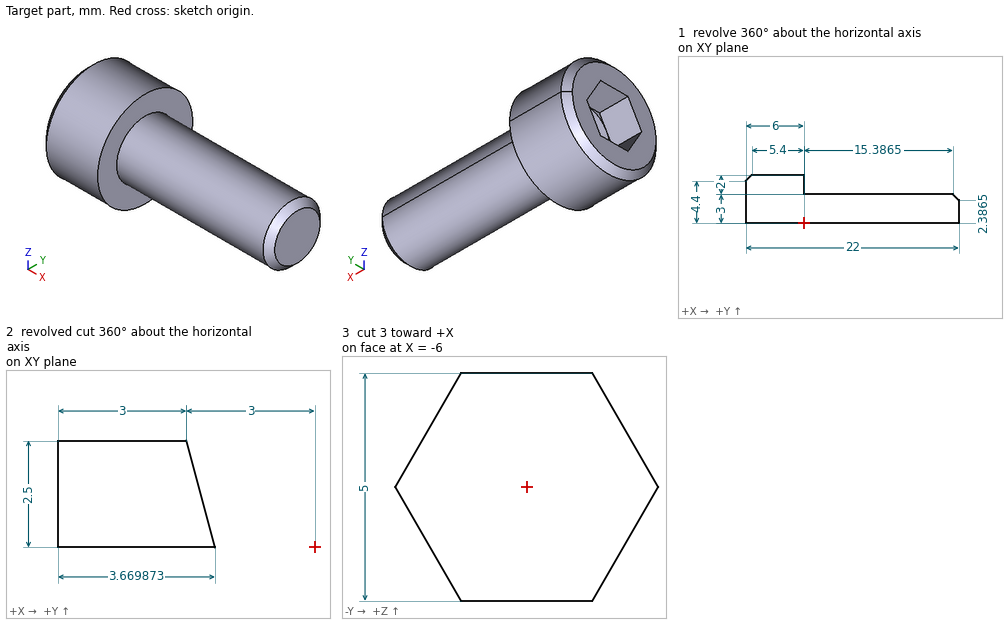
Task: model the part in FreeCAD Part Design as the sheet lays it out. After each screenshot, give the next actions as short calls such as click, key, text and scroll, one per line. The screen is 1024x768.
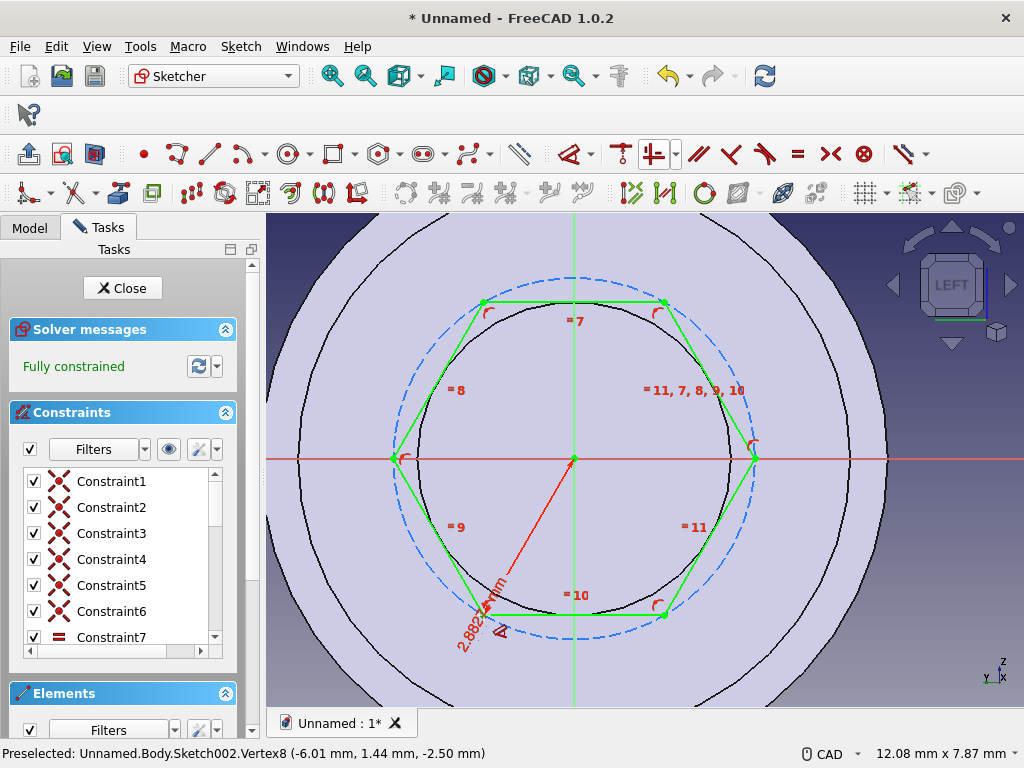
click(665, 302)
click(747, 349)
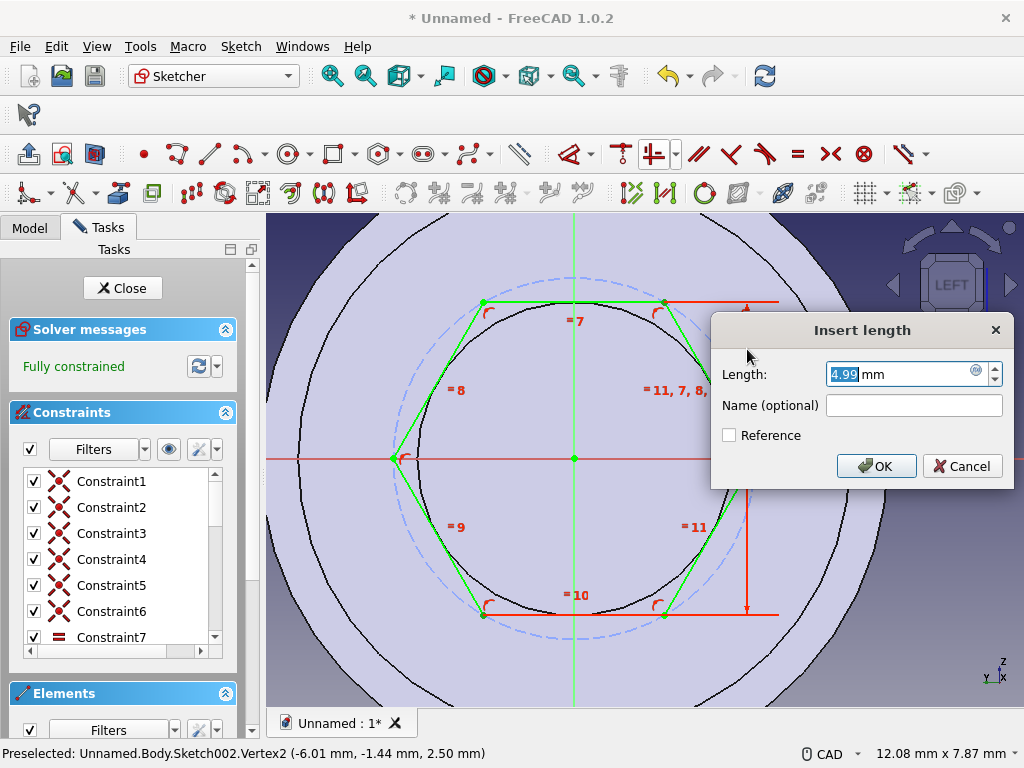
text(5)
key(Return)
key(Escape)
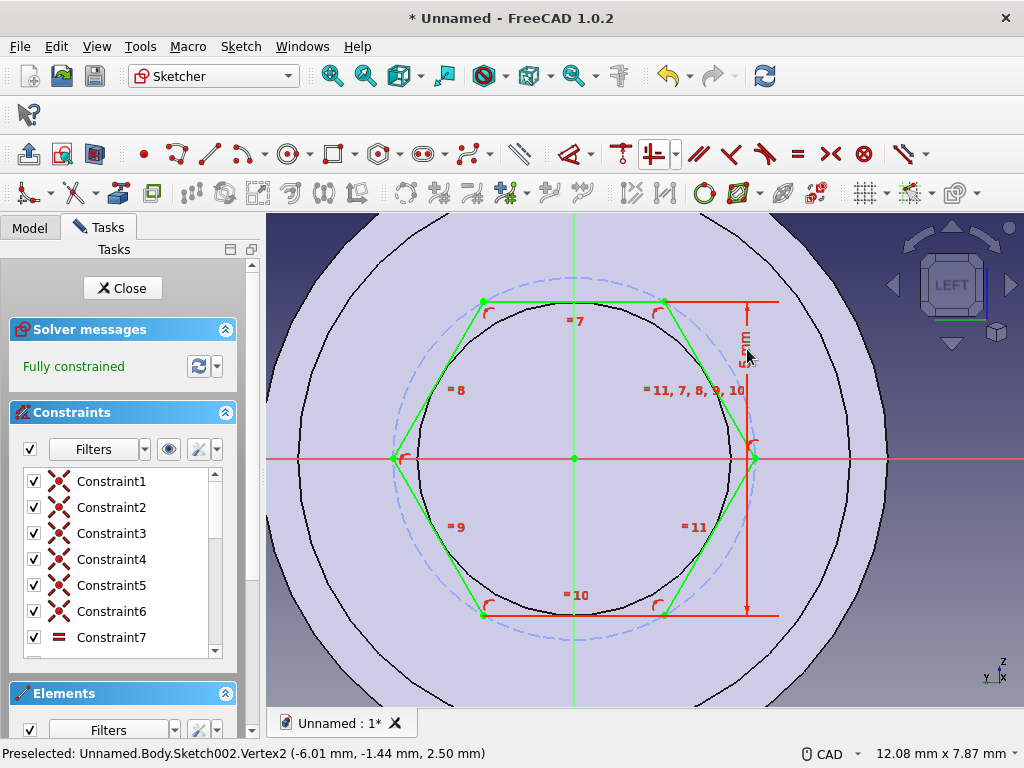
click(123, 288)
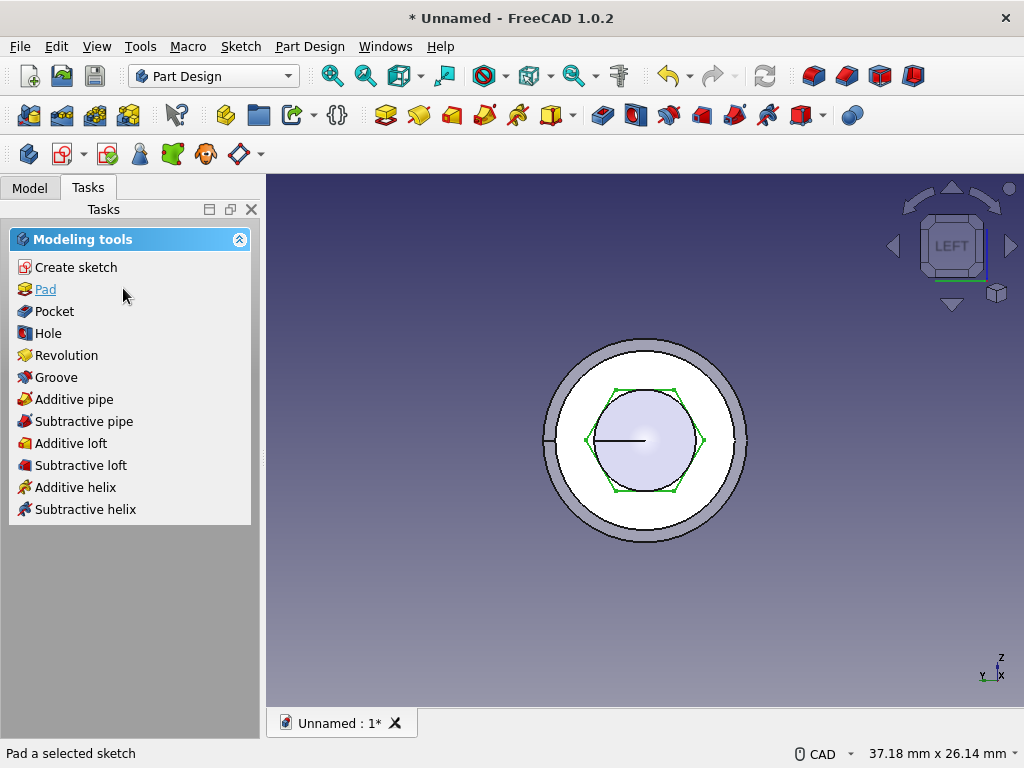
click(603, 116)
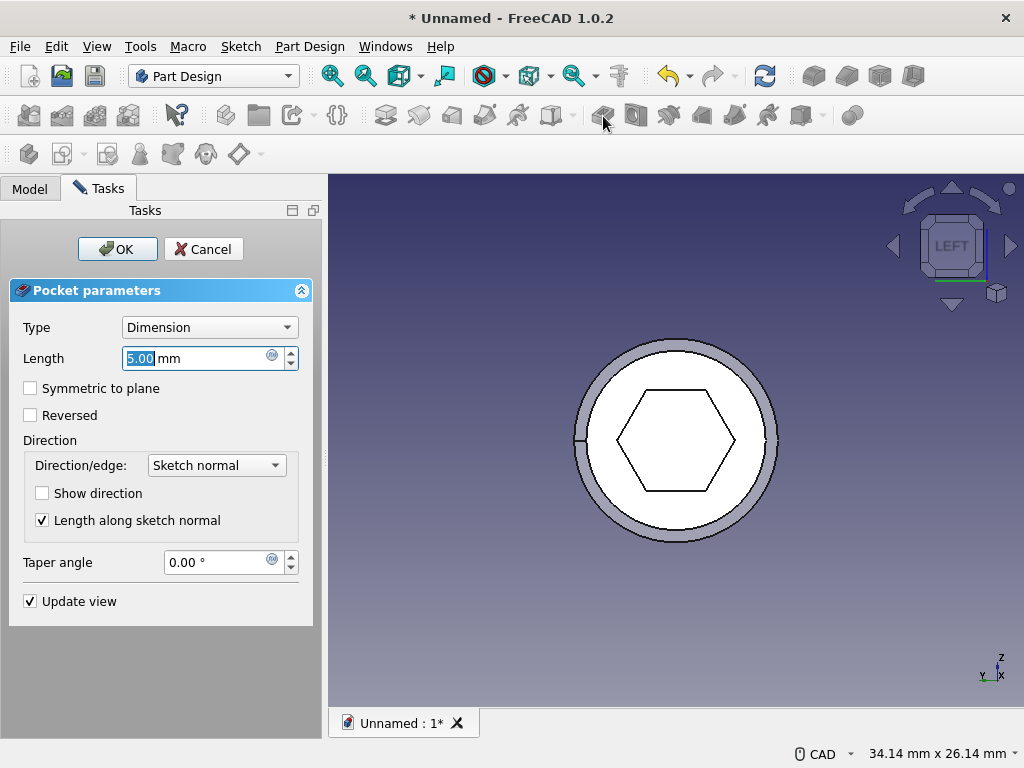
text(3)
key(Tab)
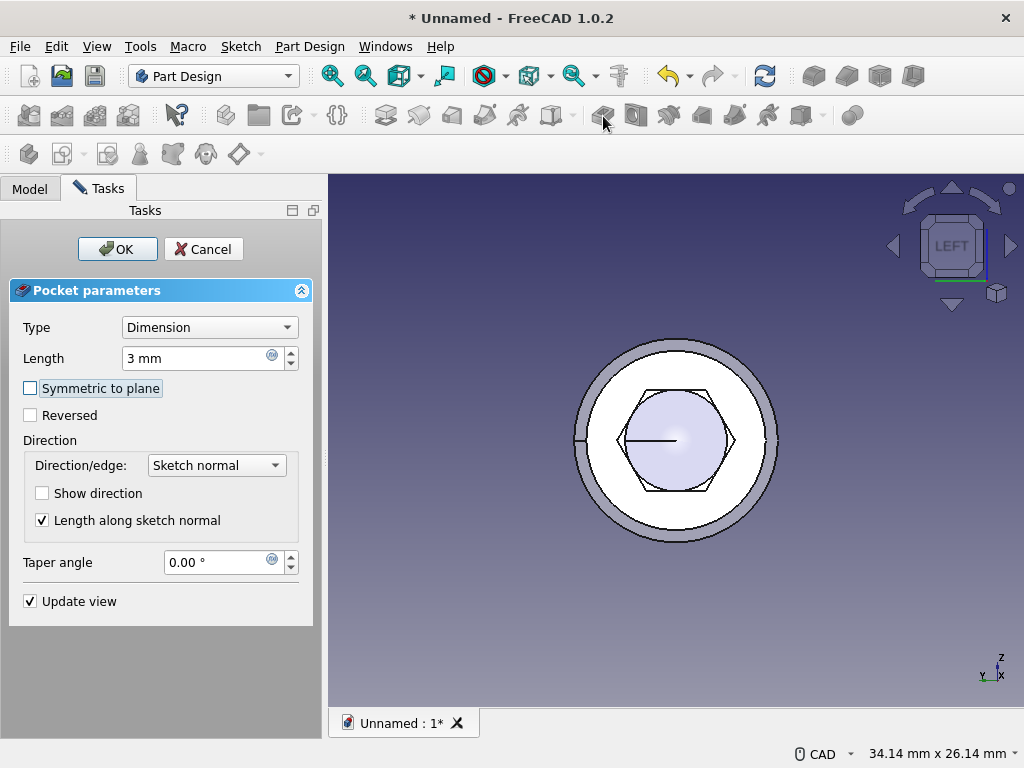
click(118, 249)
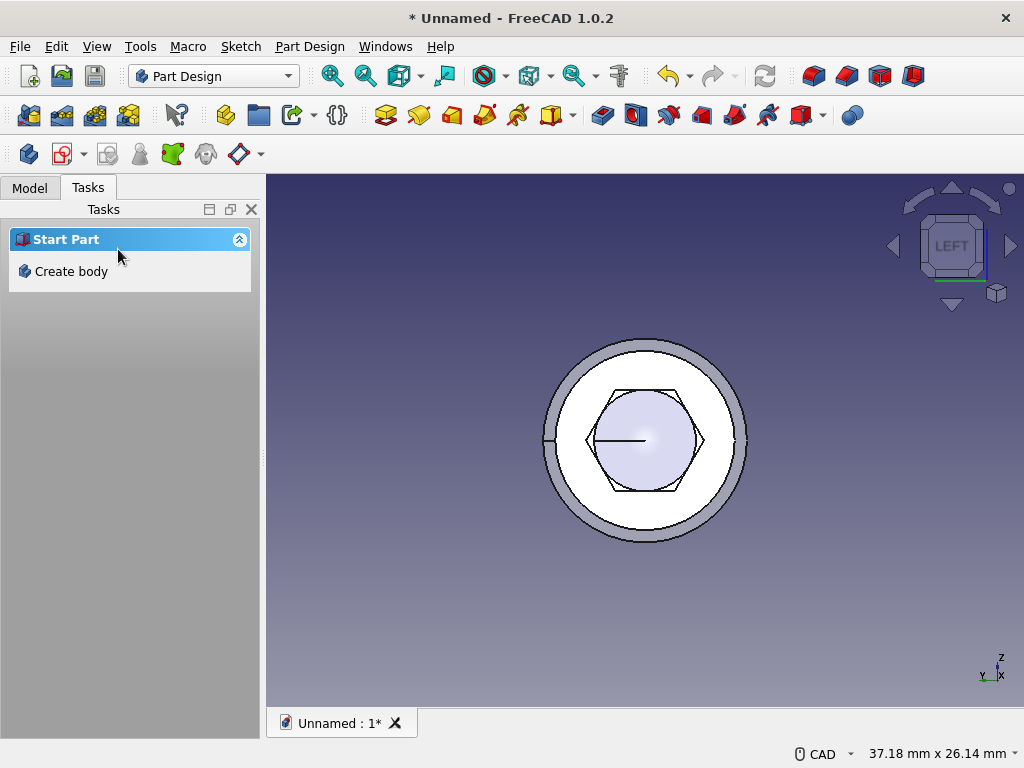
key(0)